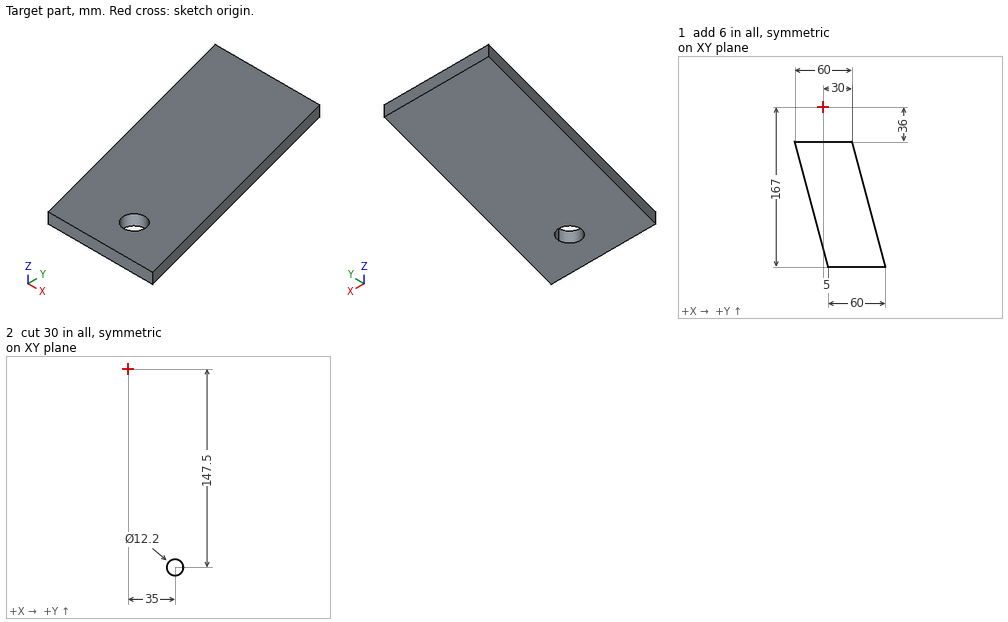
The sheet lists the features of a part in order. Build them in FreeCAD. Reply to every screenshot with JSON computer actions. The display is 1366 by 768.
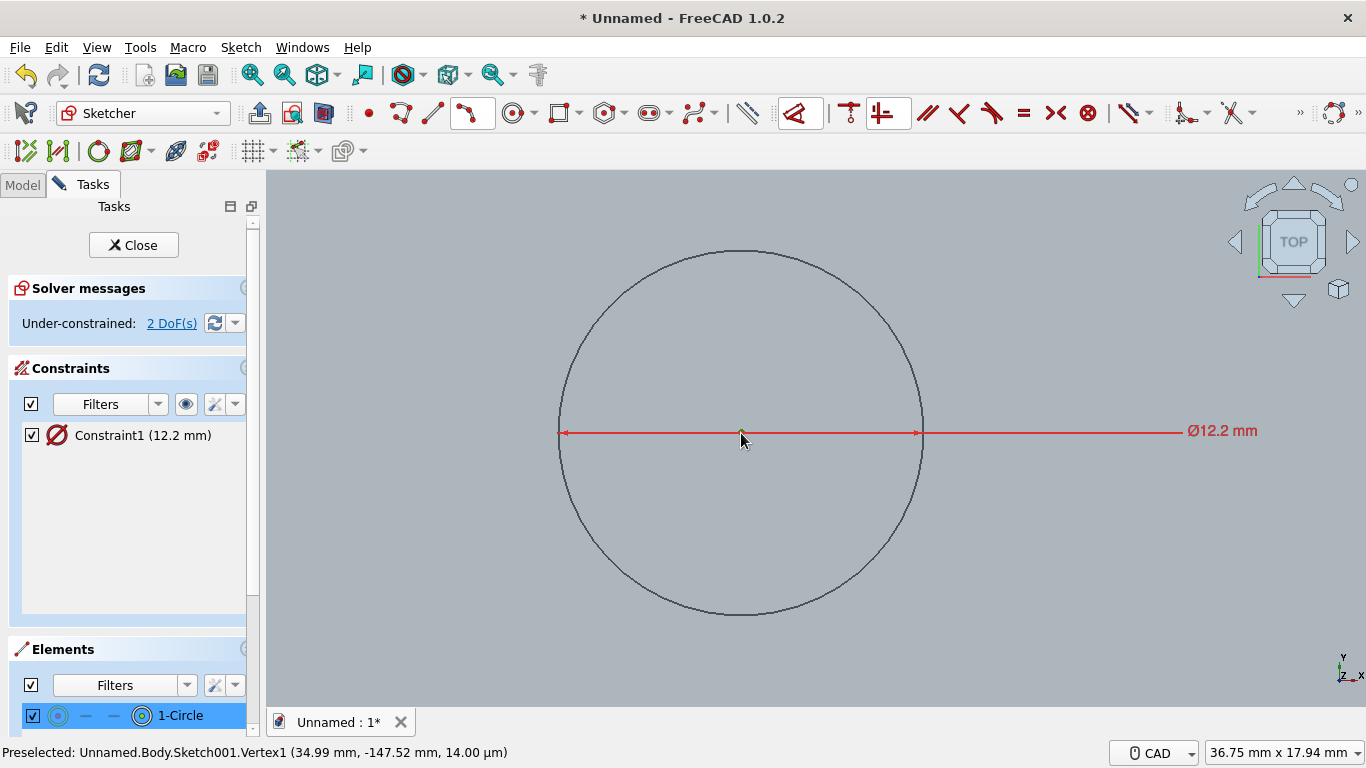
{"action": "left_click", "coordinate": [818, 114]}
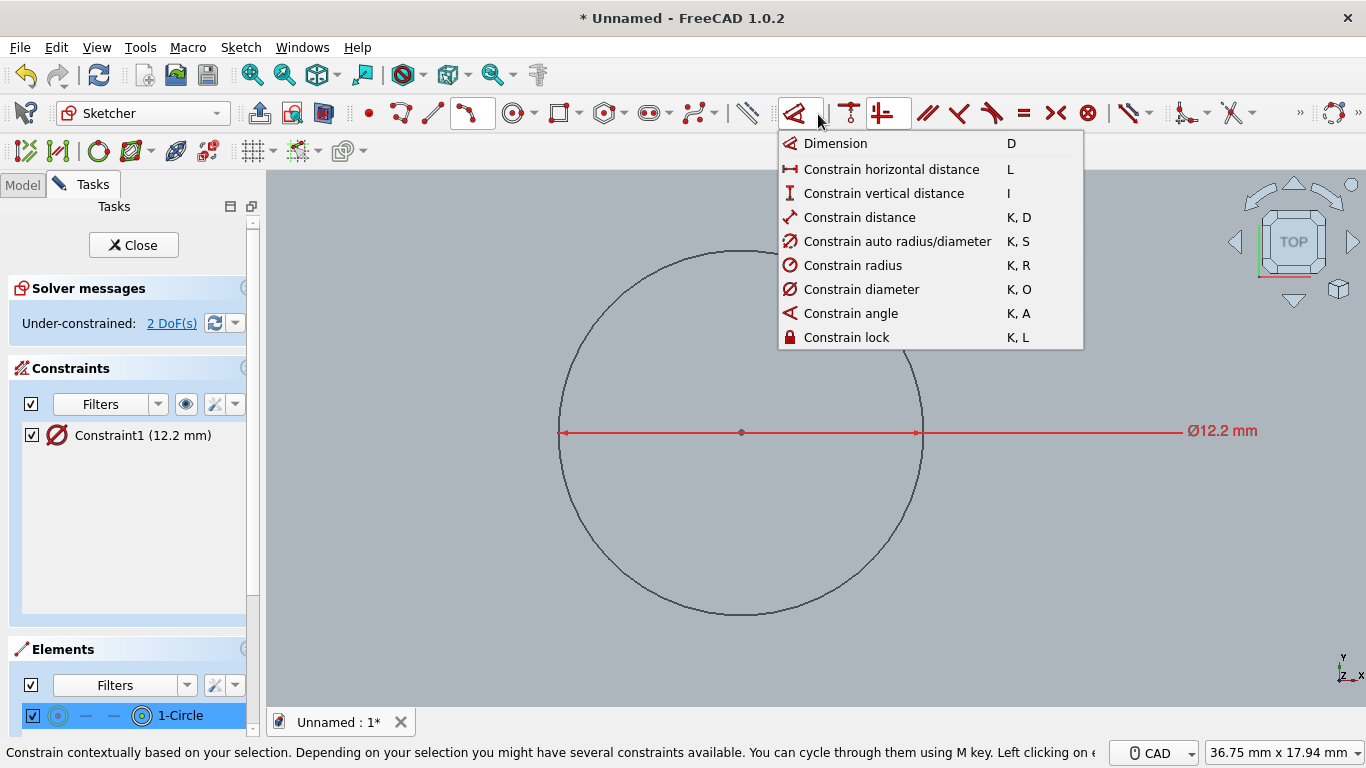
{"action": "left_click", "coordinate": [931, 169]}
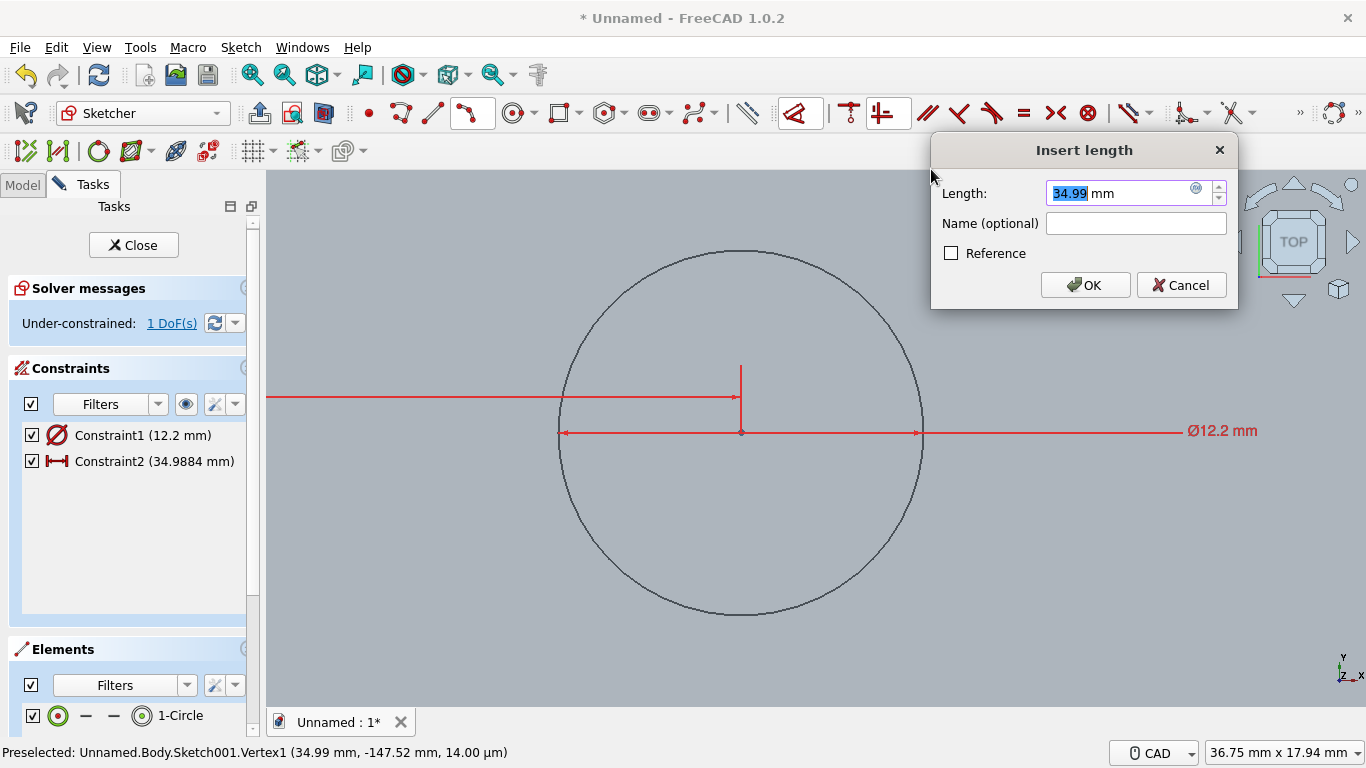
{"action": "type", "text": "35"}
{"action": "key", "text": "Return"}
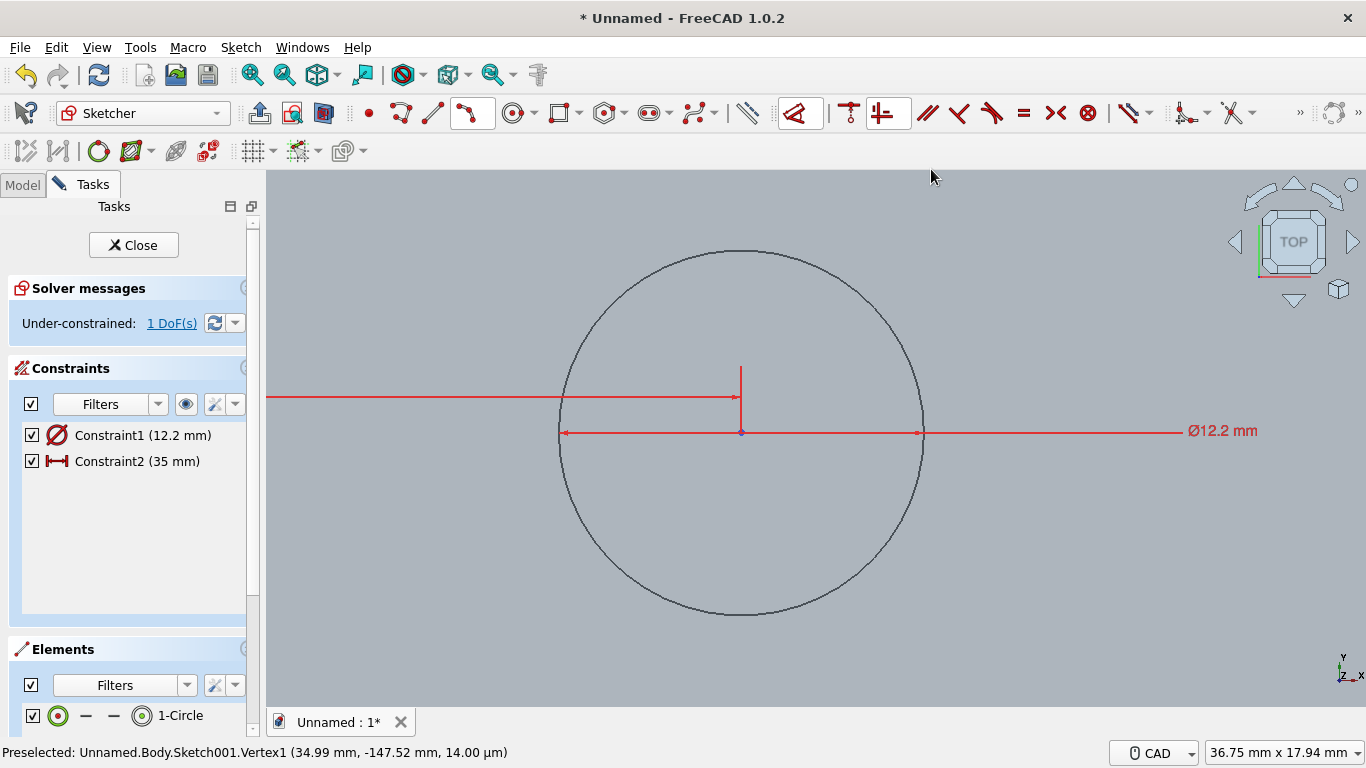
{"action": "left_click", "coordinate": [741, 433]}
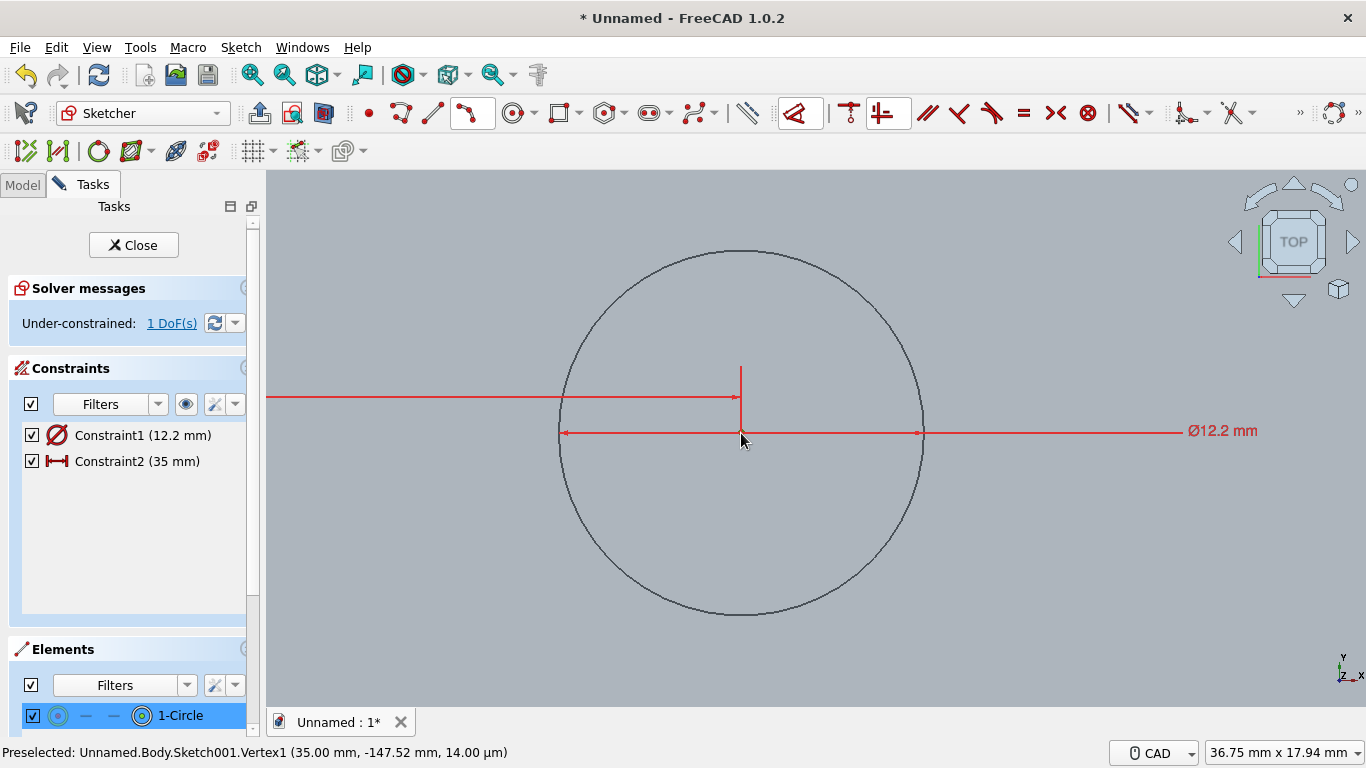
{"action": "left_click", "coordinate": [818, 114]}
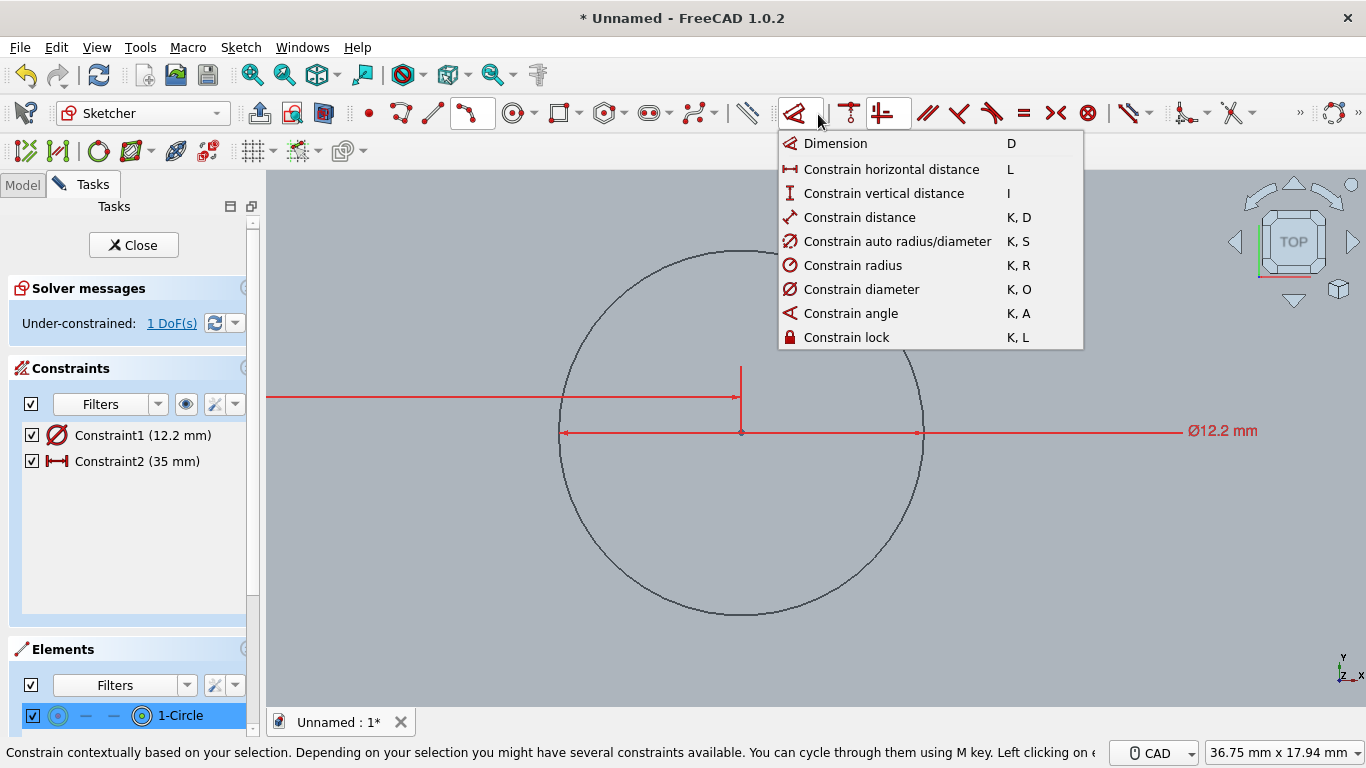
{"action": "left_click", "coordinate": [931, 193]}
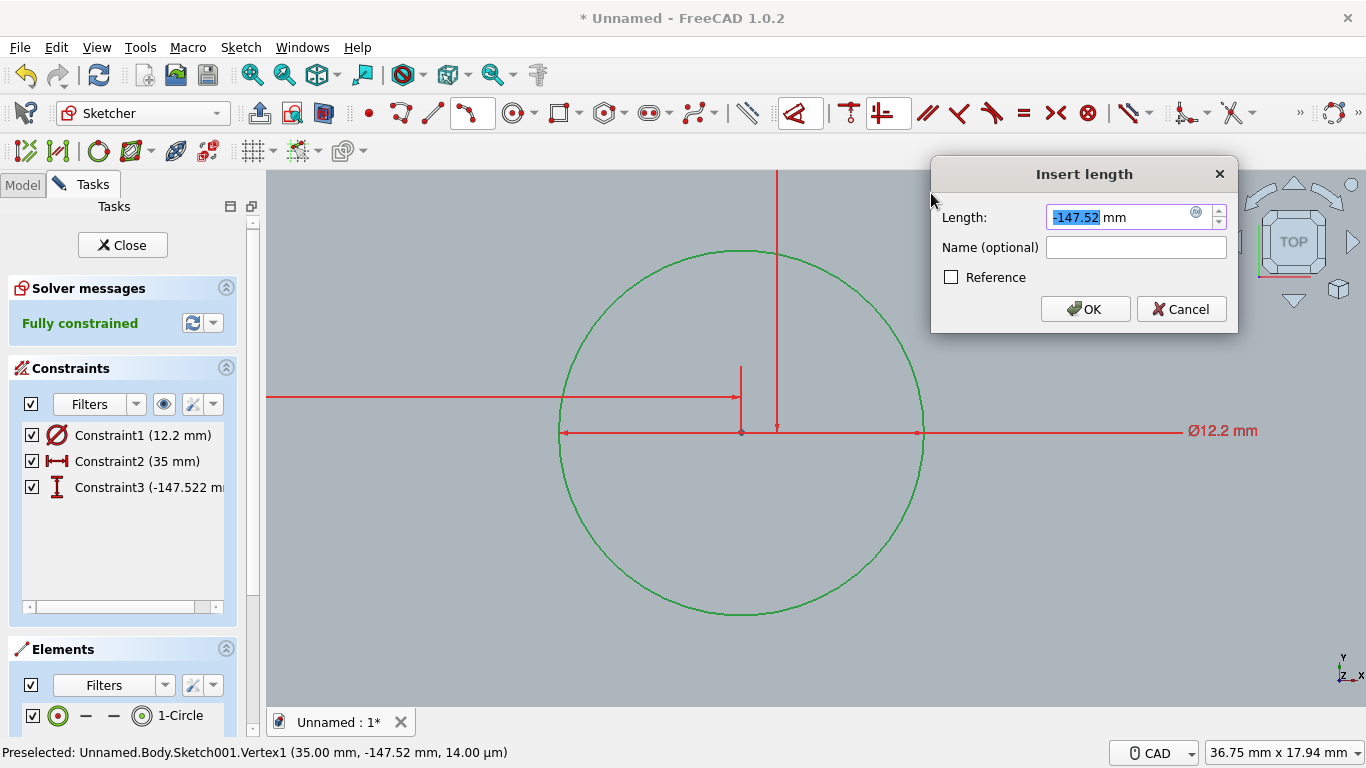
{"action": "type", "text": "-147.5"}
{"action": "key", "text": "Return"}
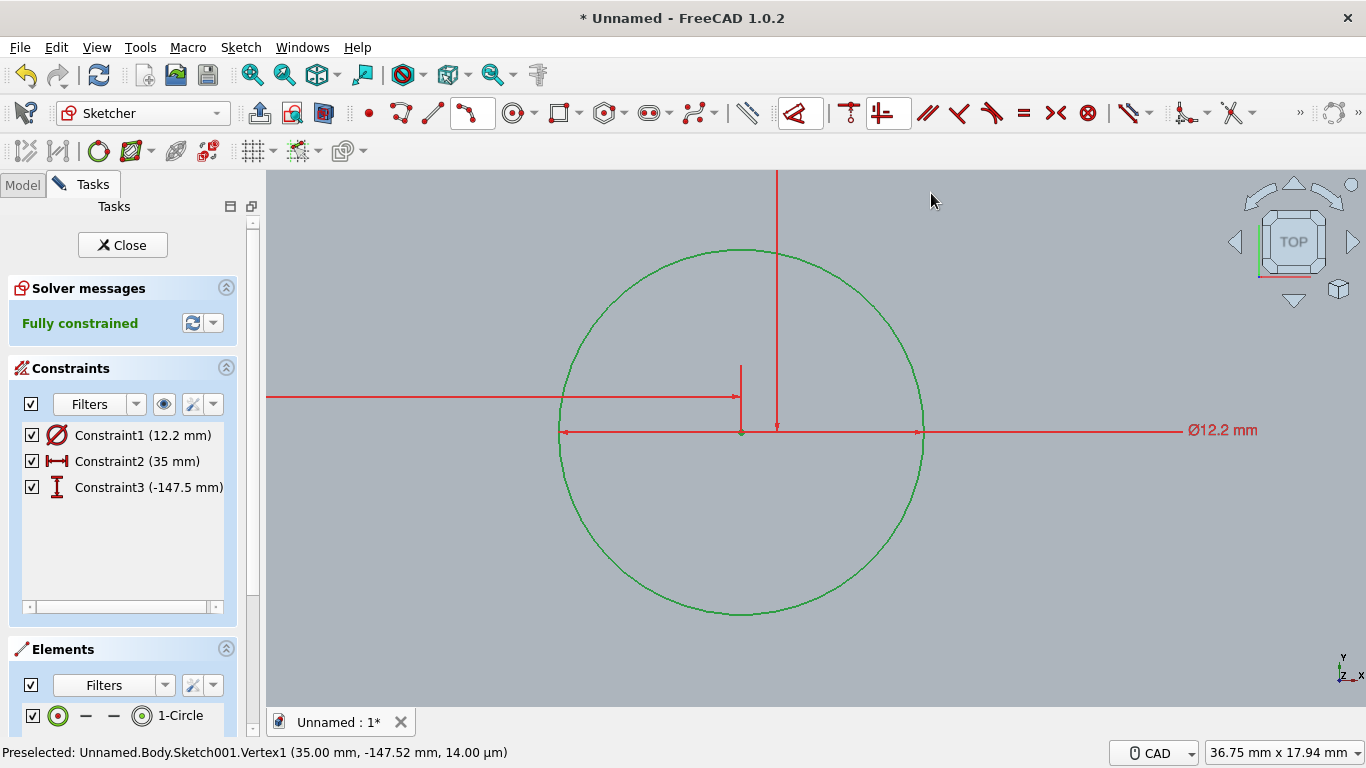
{"action": "left_click", "coordinate": [123, 245]}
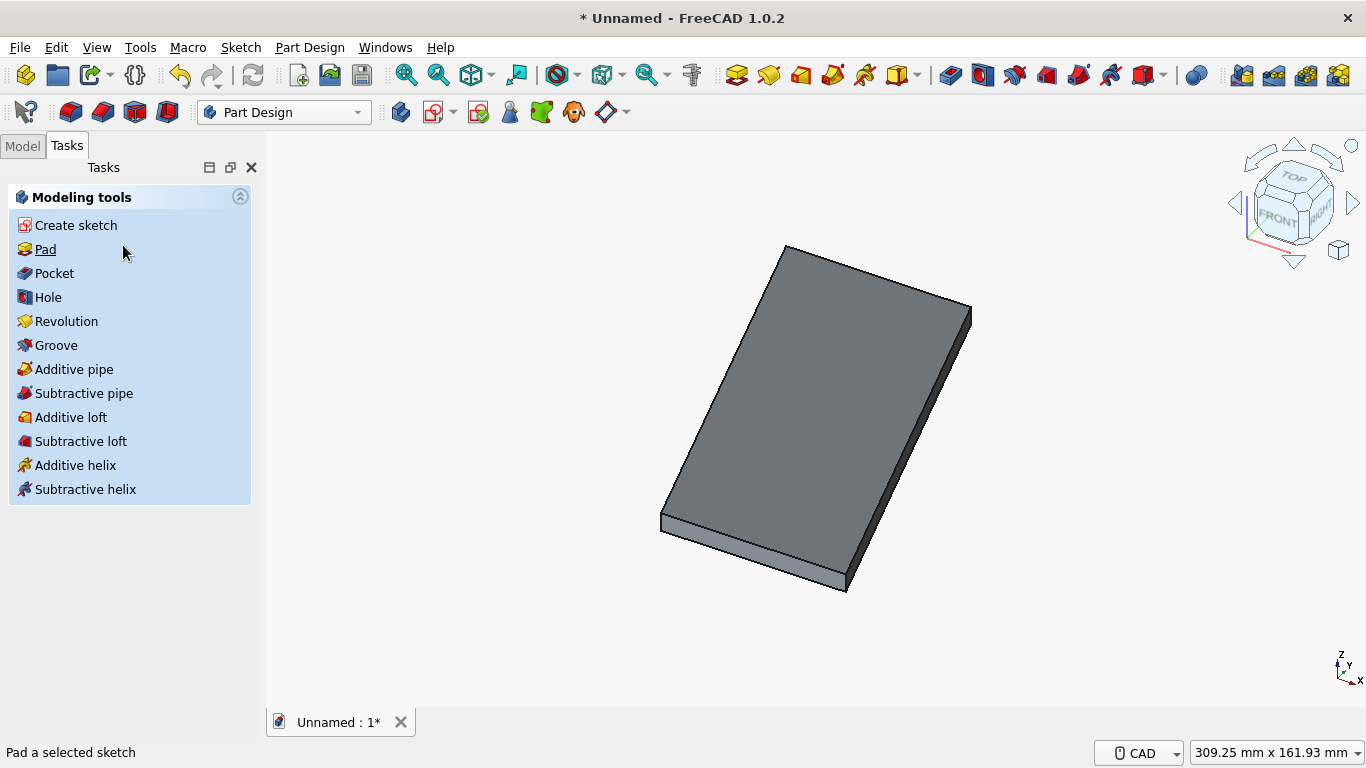
{"action": "left_click", "coordinate": [952, 76]}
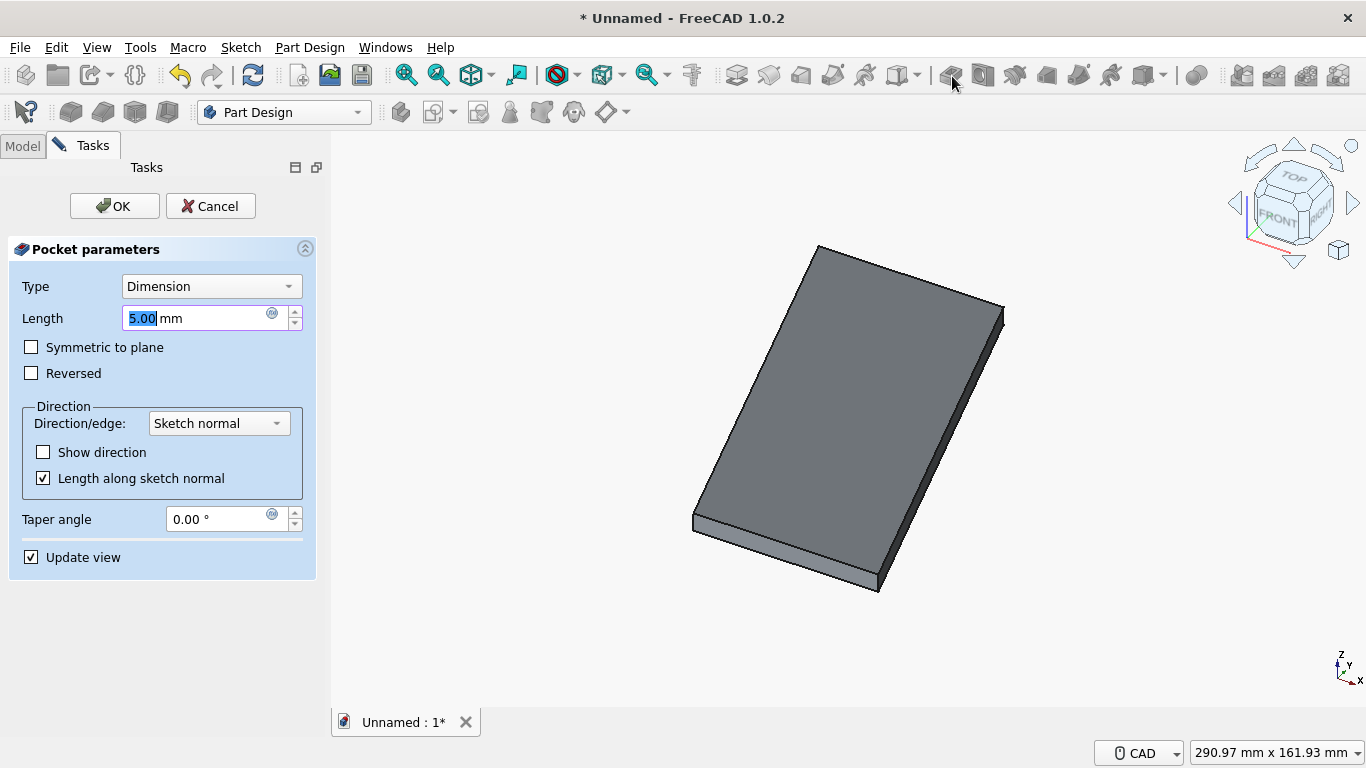
{"action": "type", "text": "30"}
{"action": "key", "text": "Tab"}